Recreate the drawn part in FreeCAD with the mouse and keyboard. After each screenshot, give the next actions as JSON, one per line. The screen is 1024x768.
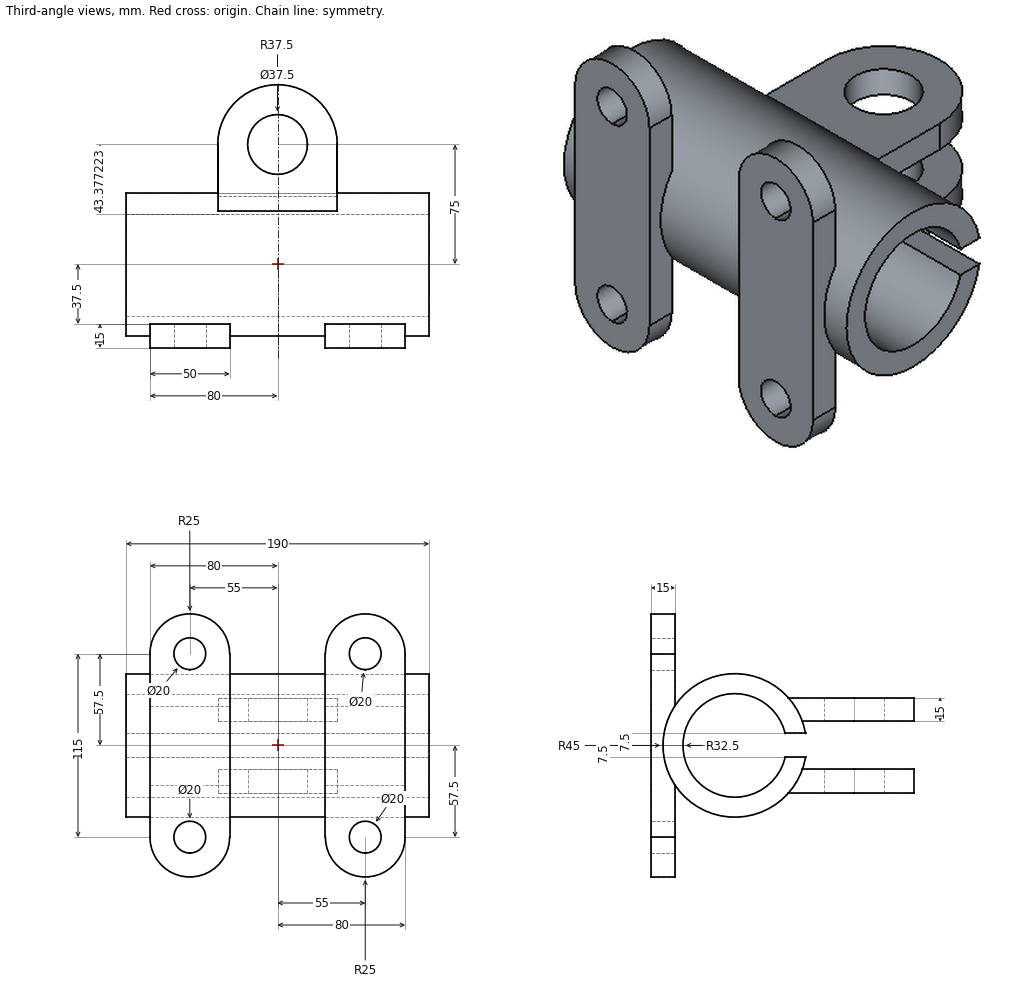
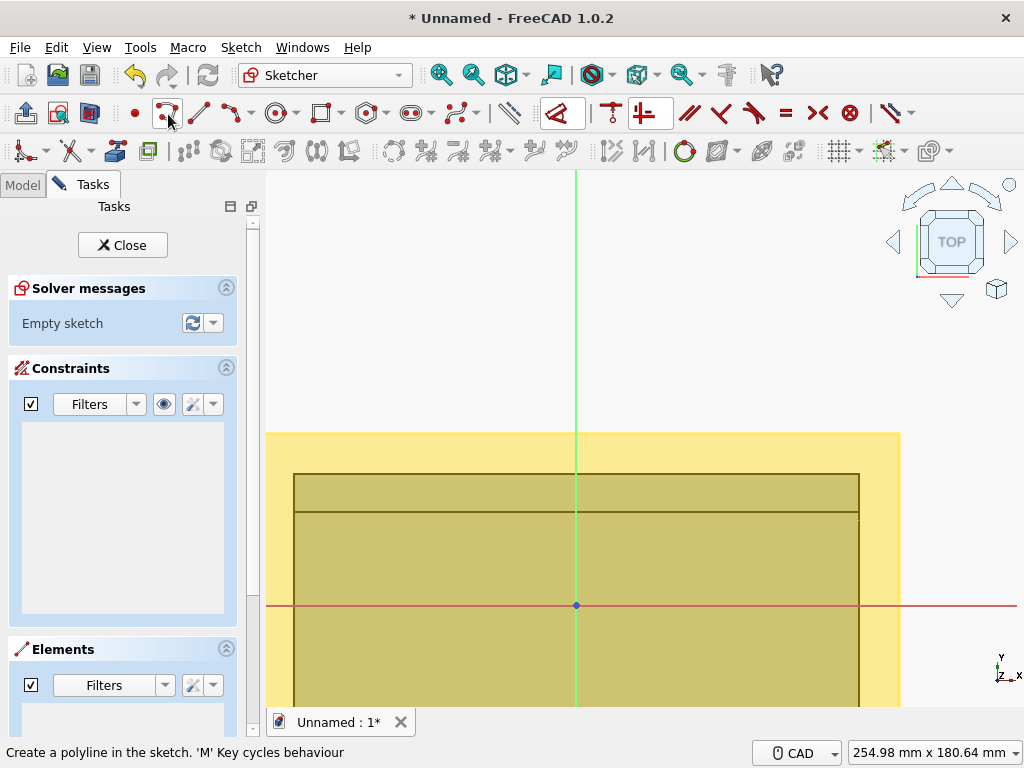
{"action": "left_click", "coordinate": [465, 383]}
{"action": "left_click", "coordinate": [465, 512]}
{"action": "left_click", "coordinate": [688, 512]}
{"action": "left_click", "coordinate": [688, 383]}
{"action": "right_click", "coordinate": [688, 383]}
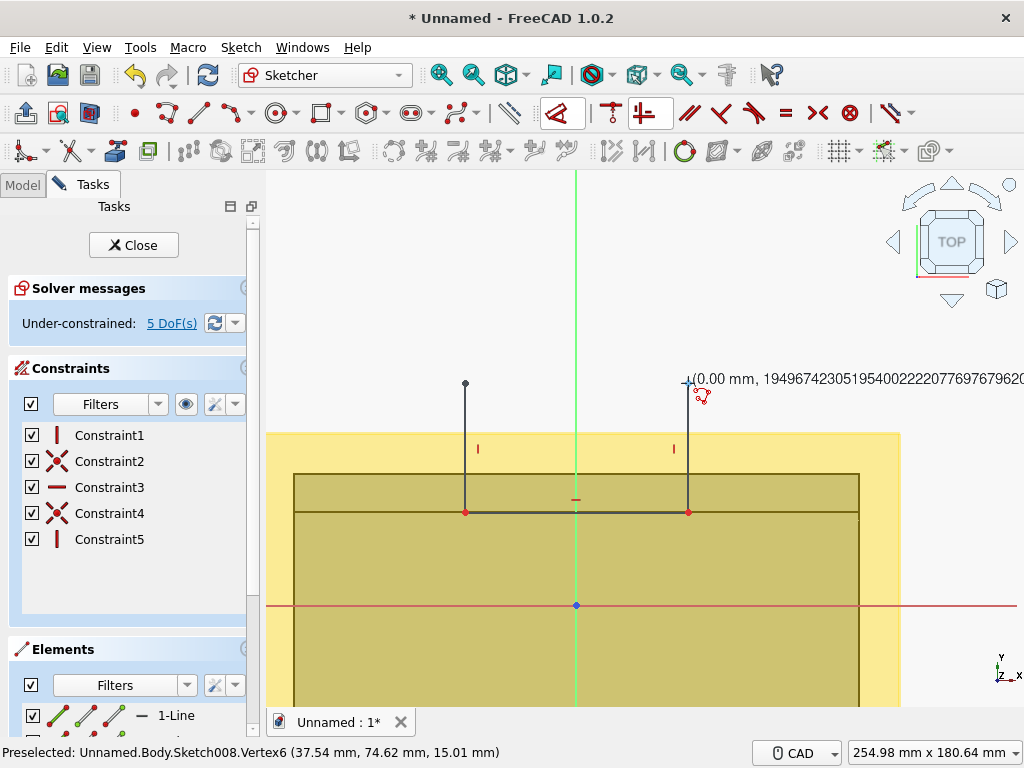
{"action": "left_click", "coordinate": [232, 114]}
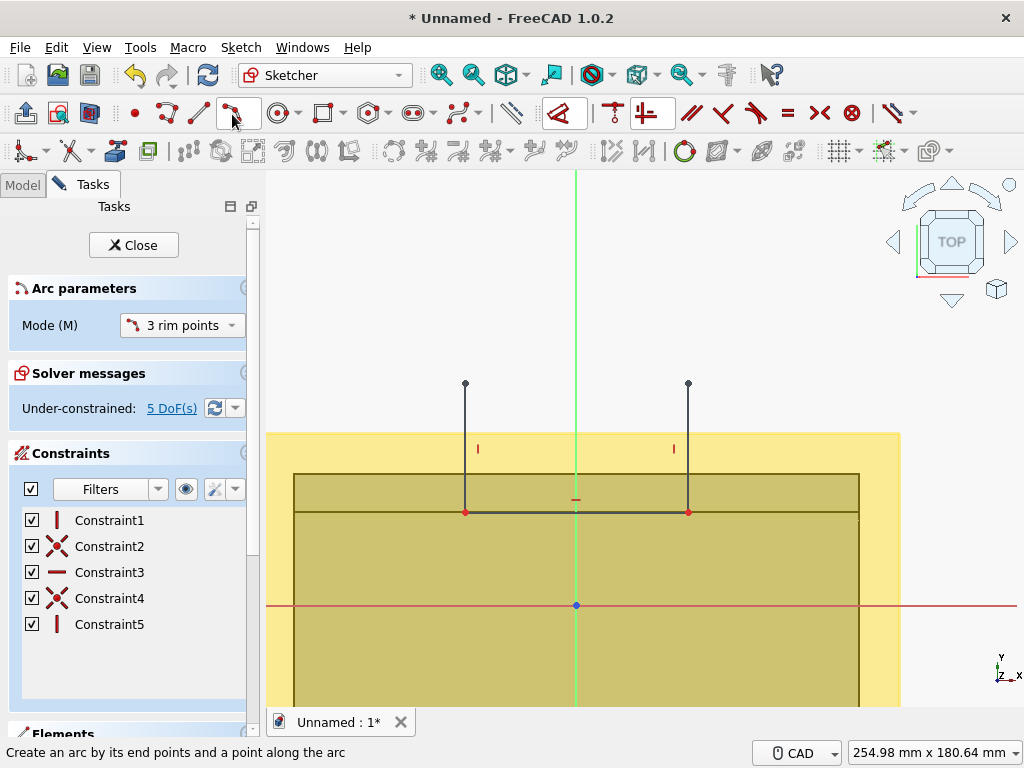
{"action": "left_click", "coordinate": [688, 384]}
{"action": "left_click", "coordinate": [465, 384]}
{"action": "left_click", "coordinate": [611, 277]}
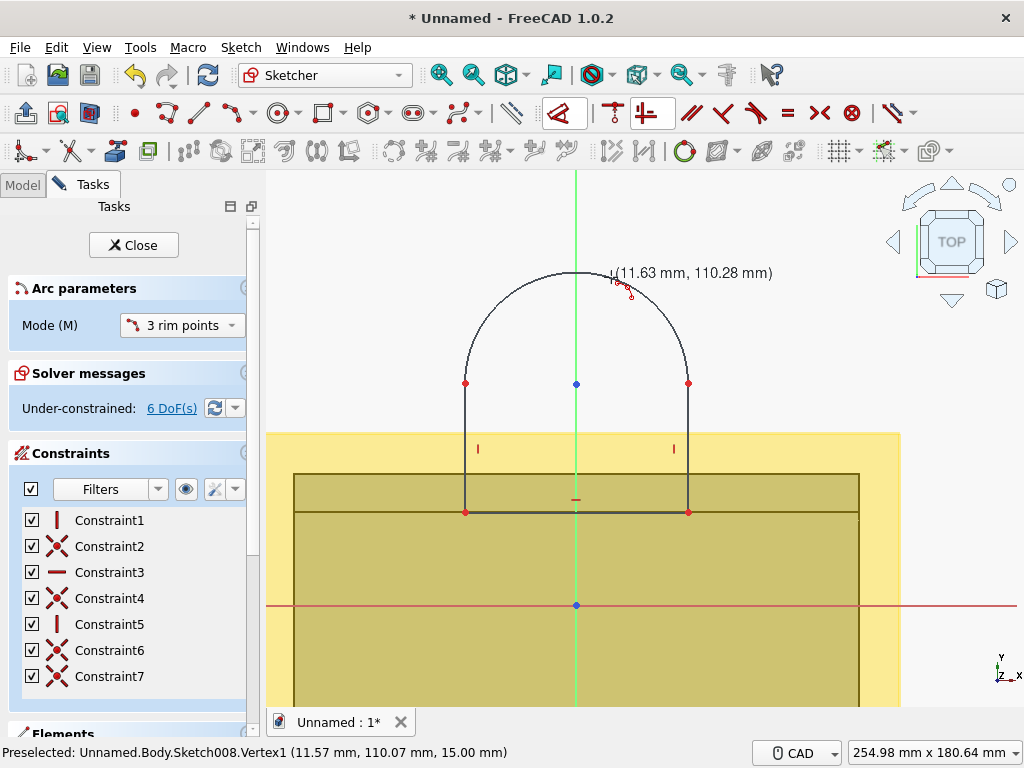
{"action": "left_click", "coordinate": [278, 114]}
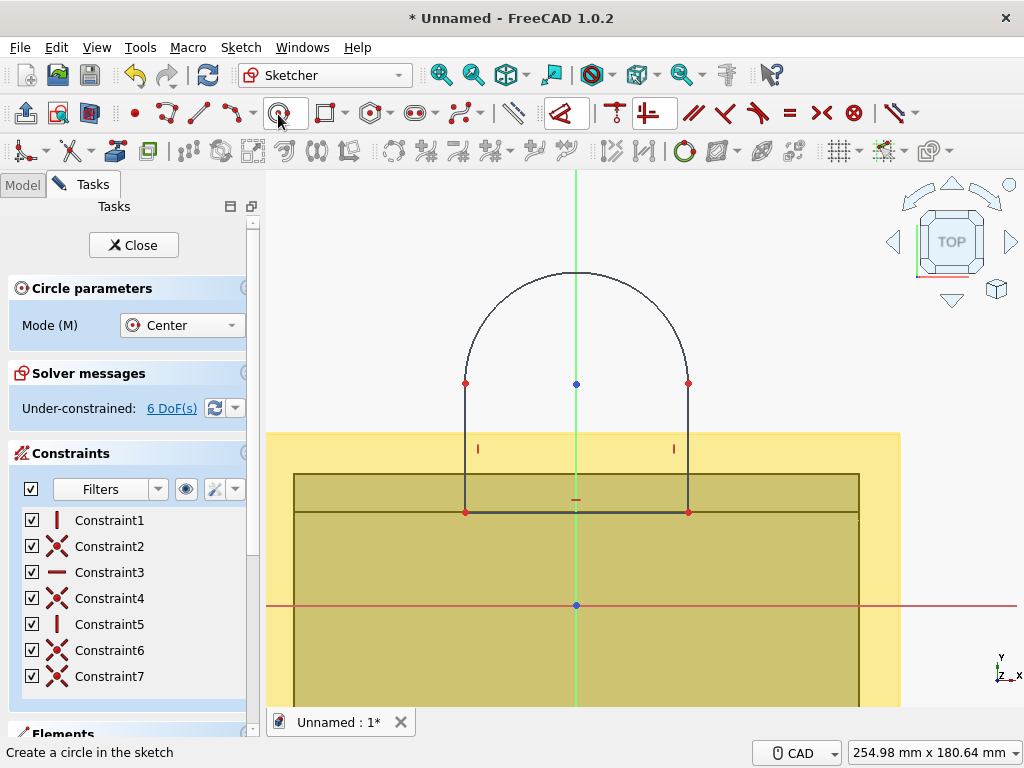
{"action": "left_click", "coordinate": [576, 383]}
{"action": "left_click", "coordinate": [616, 343]}
{"action": "key", "text": "Escape"}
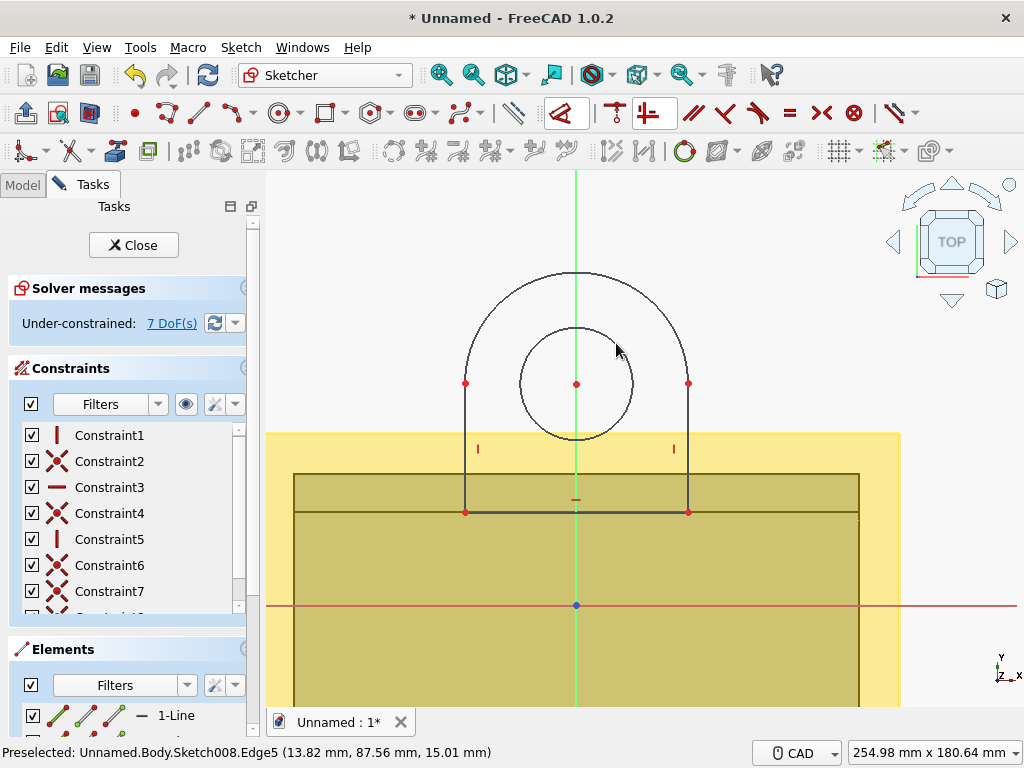
{"action": "left_click", "coordinate": [465, 423]}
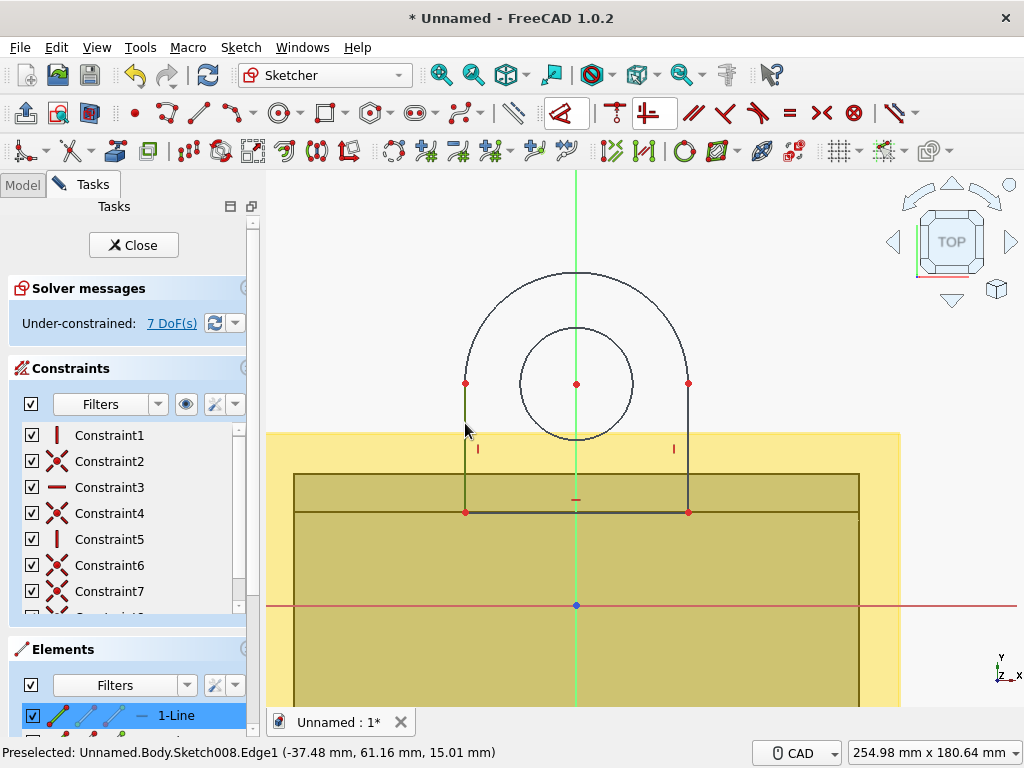
{"action": "left_click", "coordinate": [642, 294]}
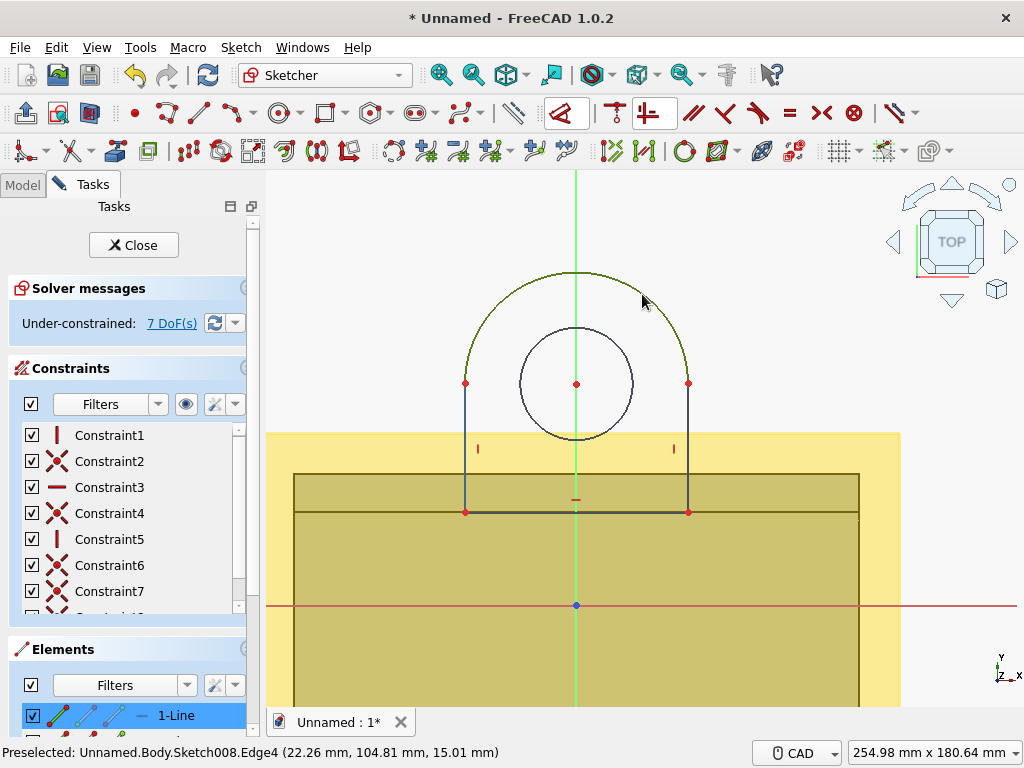
{"action": "left_click", "coordinate": [758, 114]}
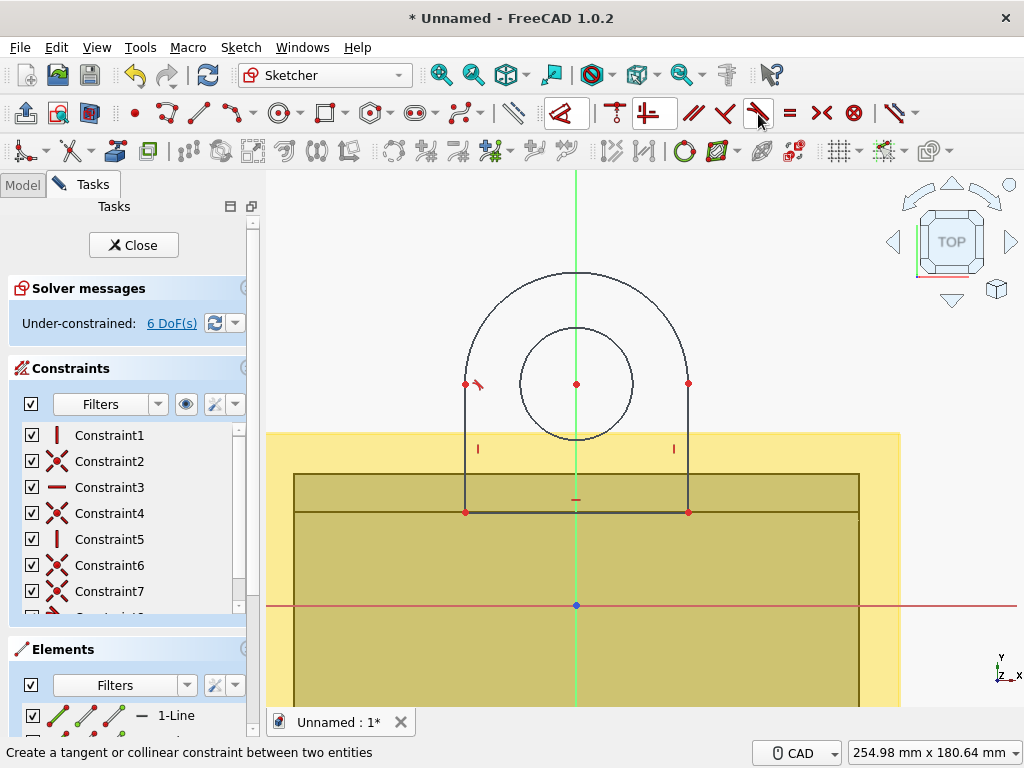
{"action": "left_click", "coordinate": [688, 474]}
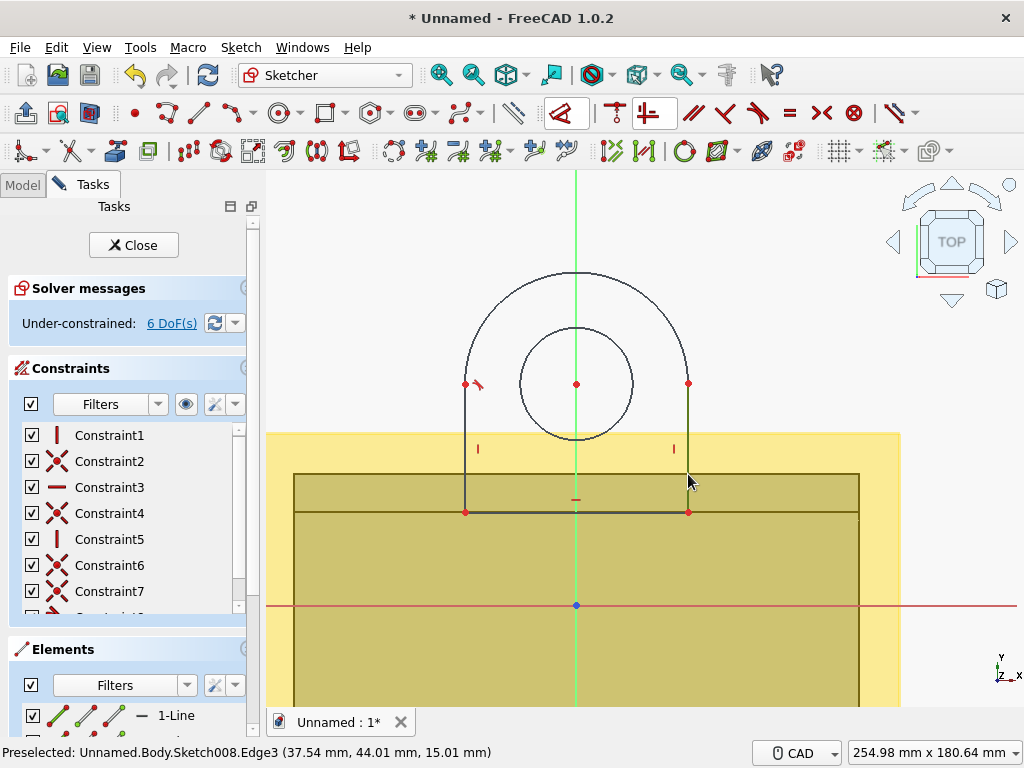
{"action": "left_click", "coordinate": [642, 294]}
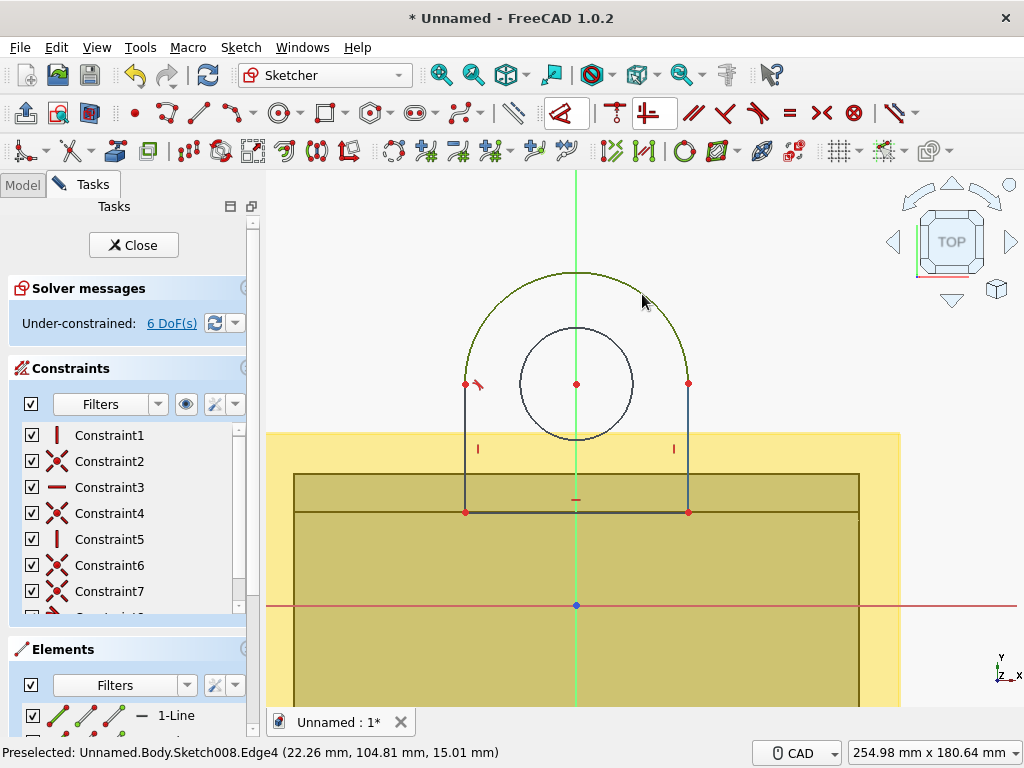
{"action": "left_click", "coordinate": [758, 114]}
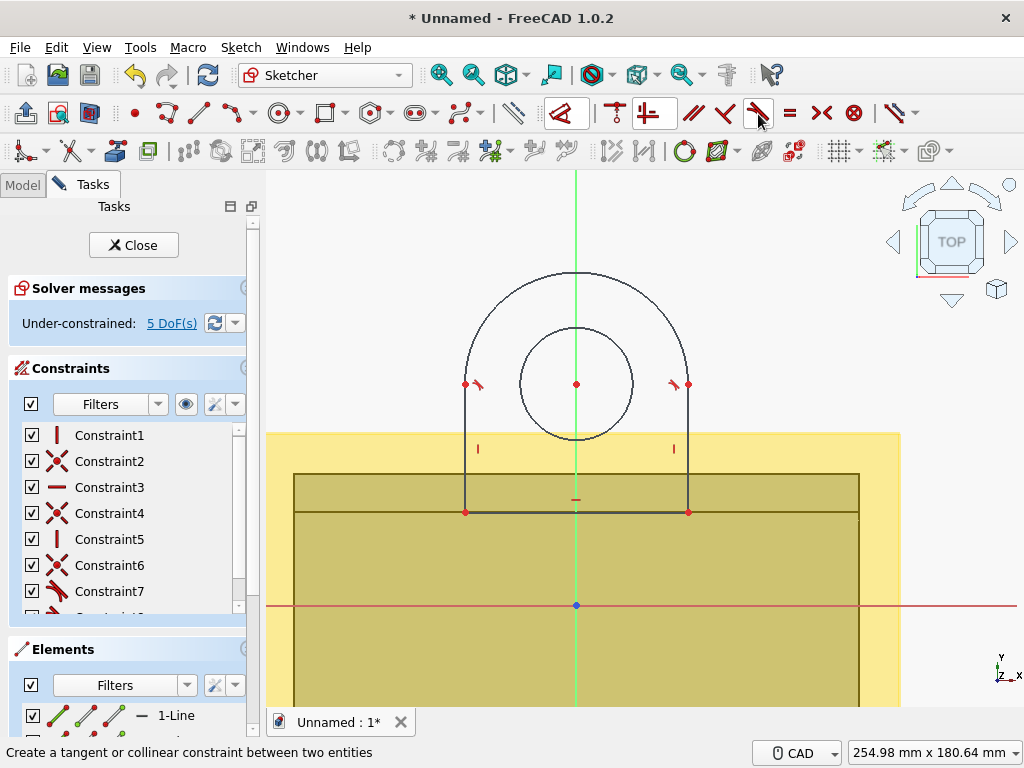
{"action": "left_click", "coordinate": [576, 384]}